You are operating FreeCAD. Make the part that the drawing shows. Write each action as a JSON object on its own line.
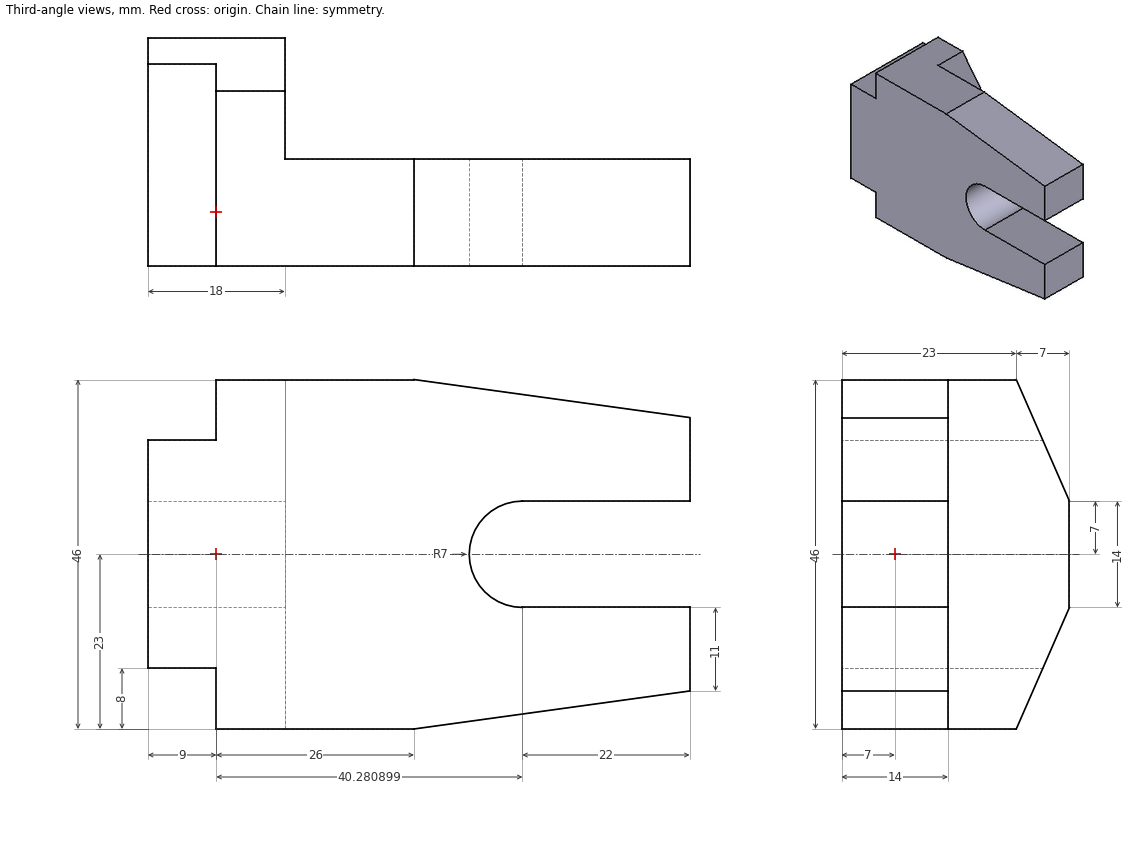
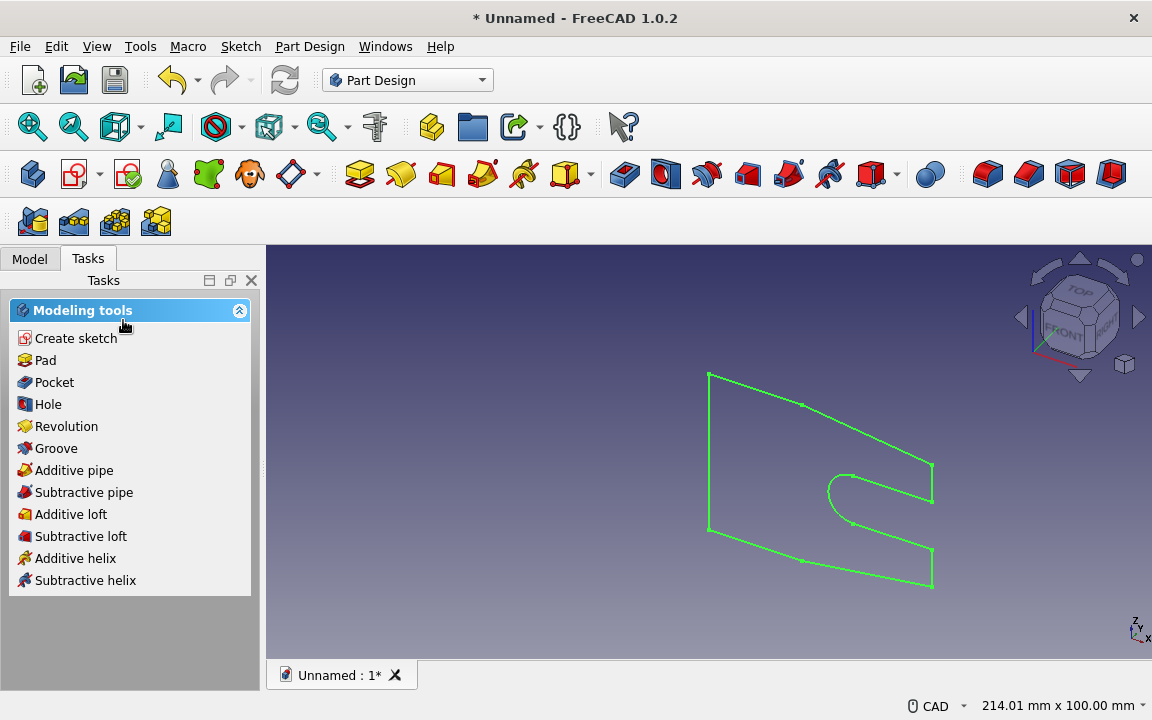
{"action": "left_click", "coordinate": [360, 174]}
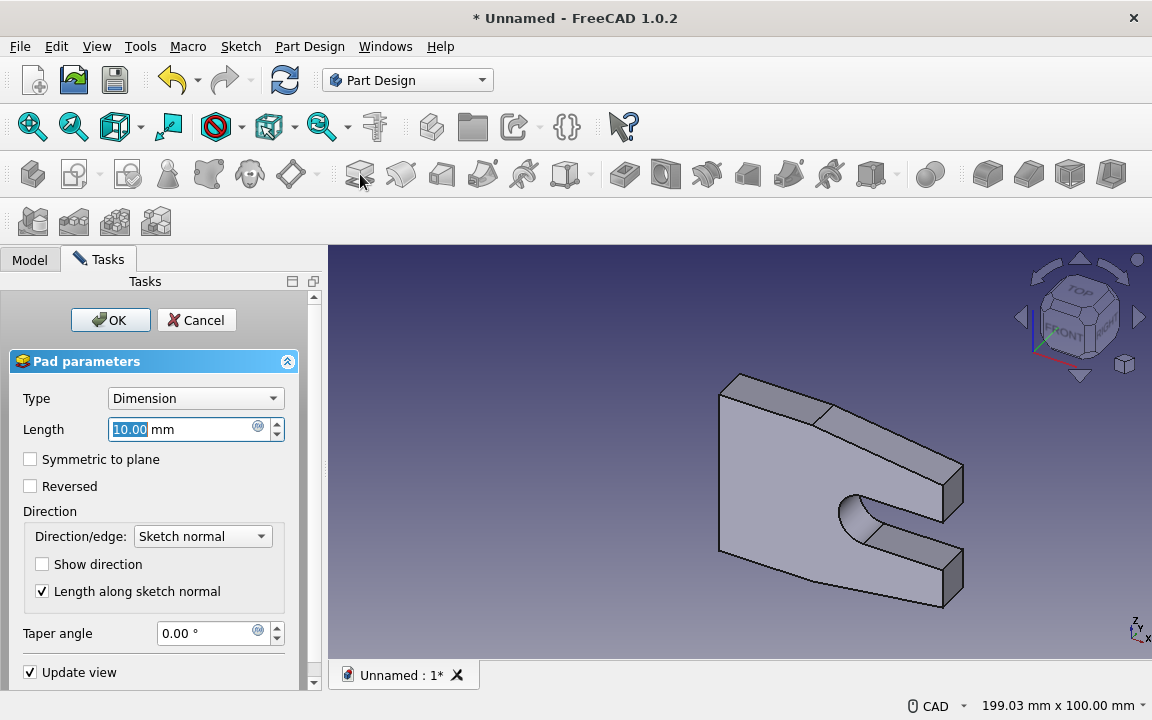
{"action": "type", "text": "14"}
{"action": "key", "text": "Tab"}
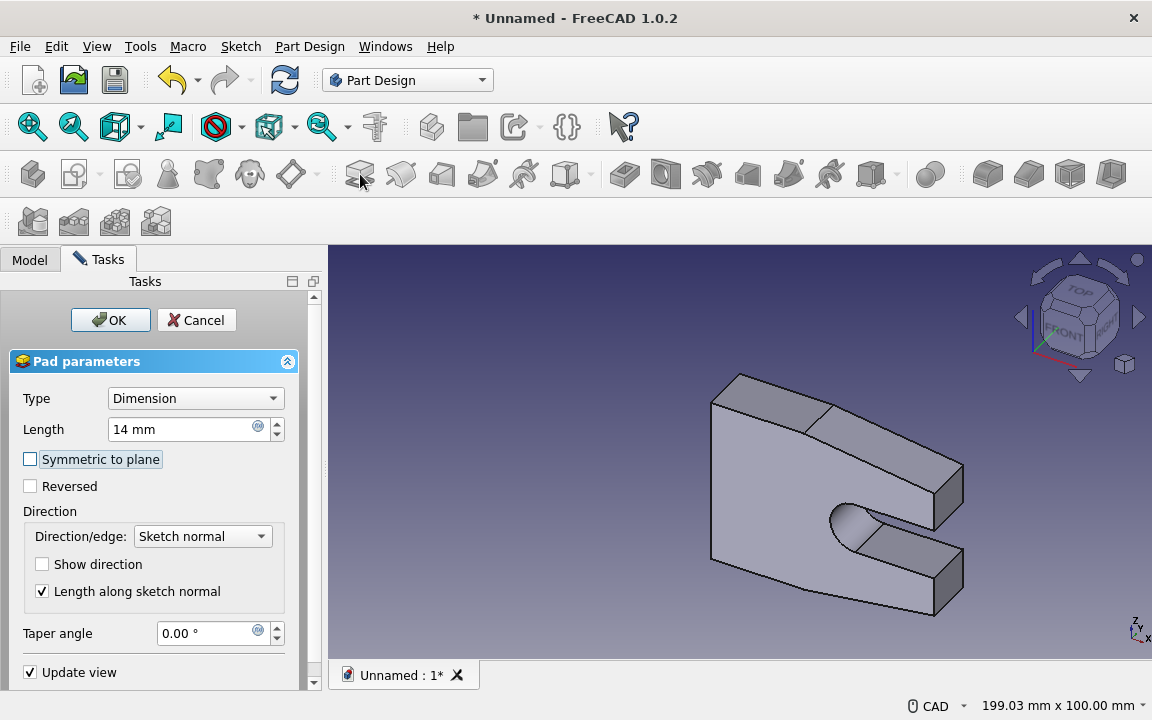
{"action": "left_click", "coordinate": [31, 459]}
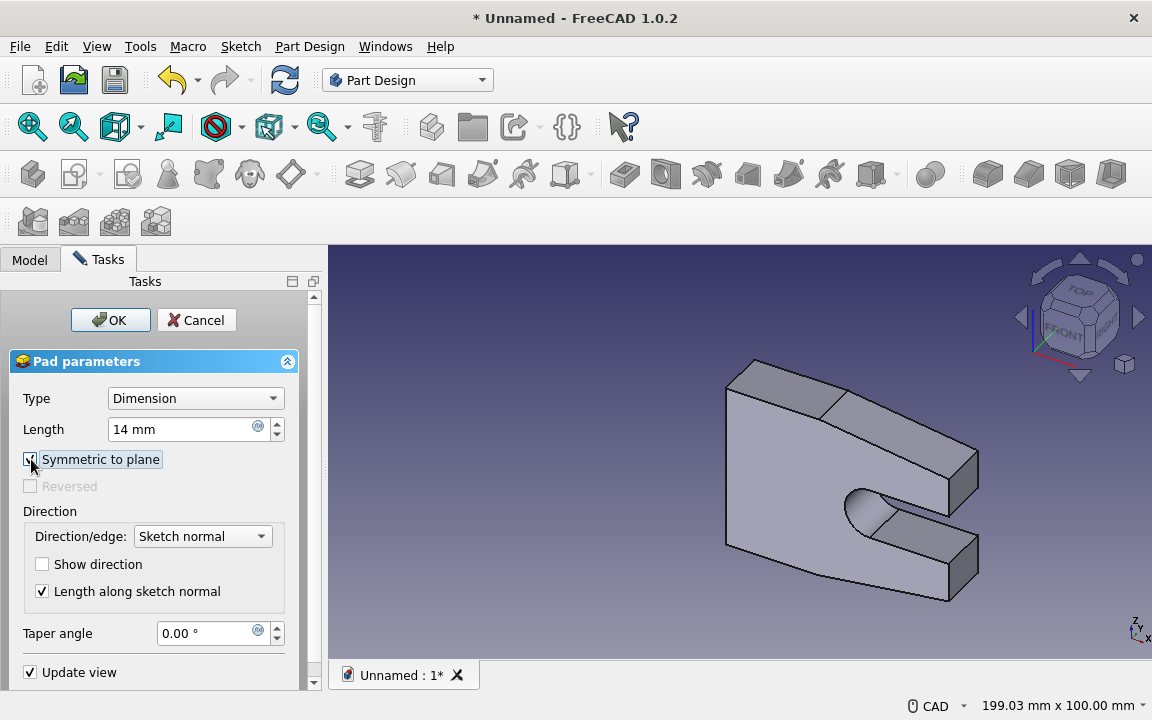
{"action": "left_click", "coordinate": [111, 320]}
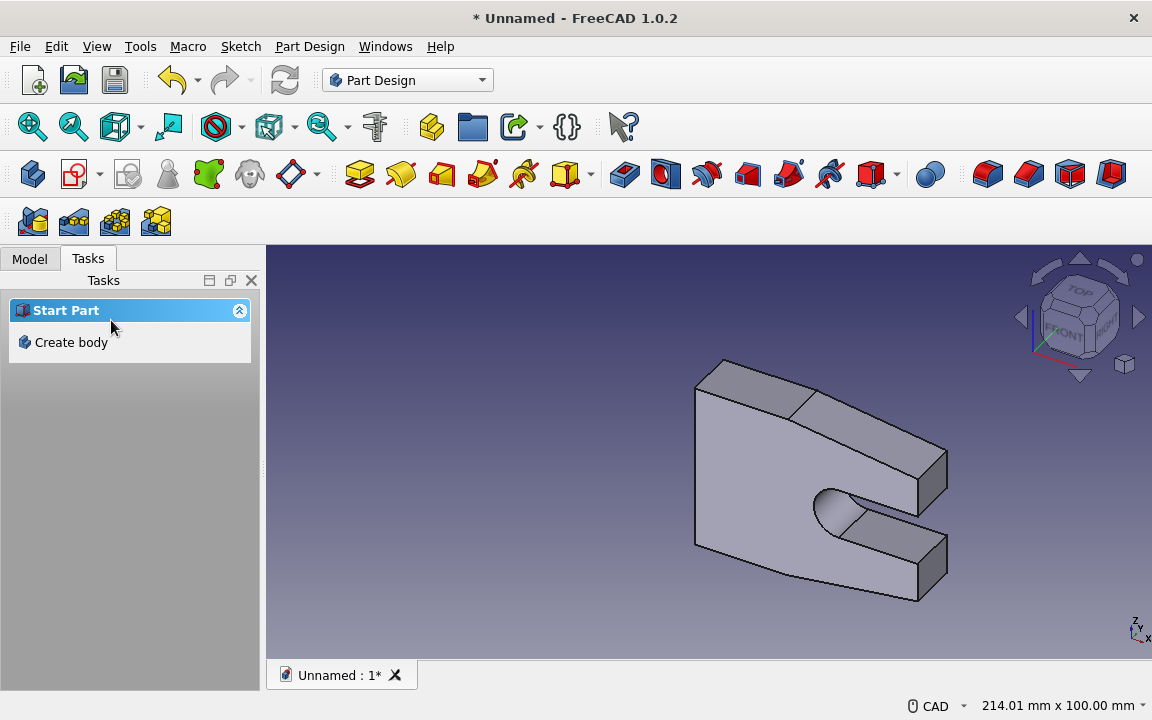
{"action": "left_click", "coordinate": [74, 174]}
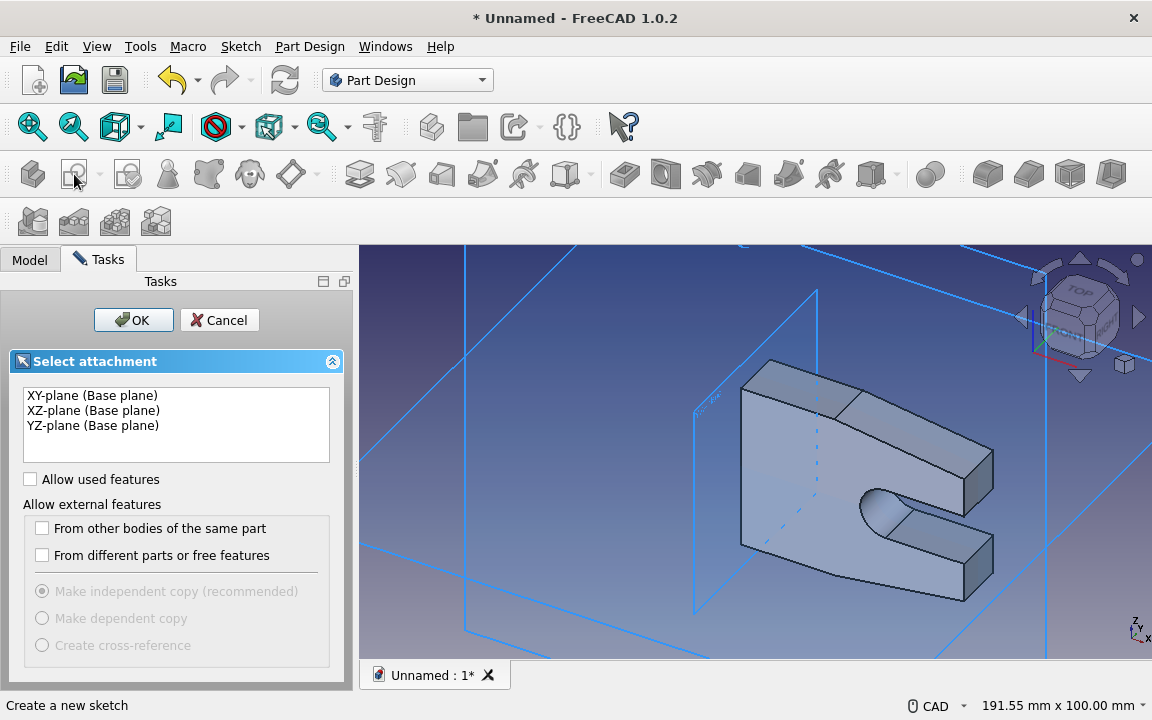
{"action": "left_click", "coordinate": [84, 426]}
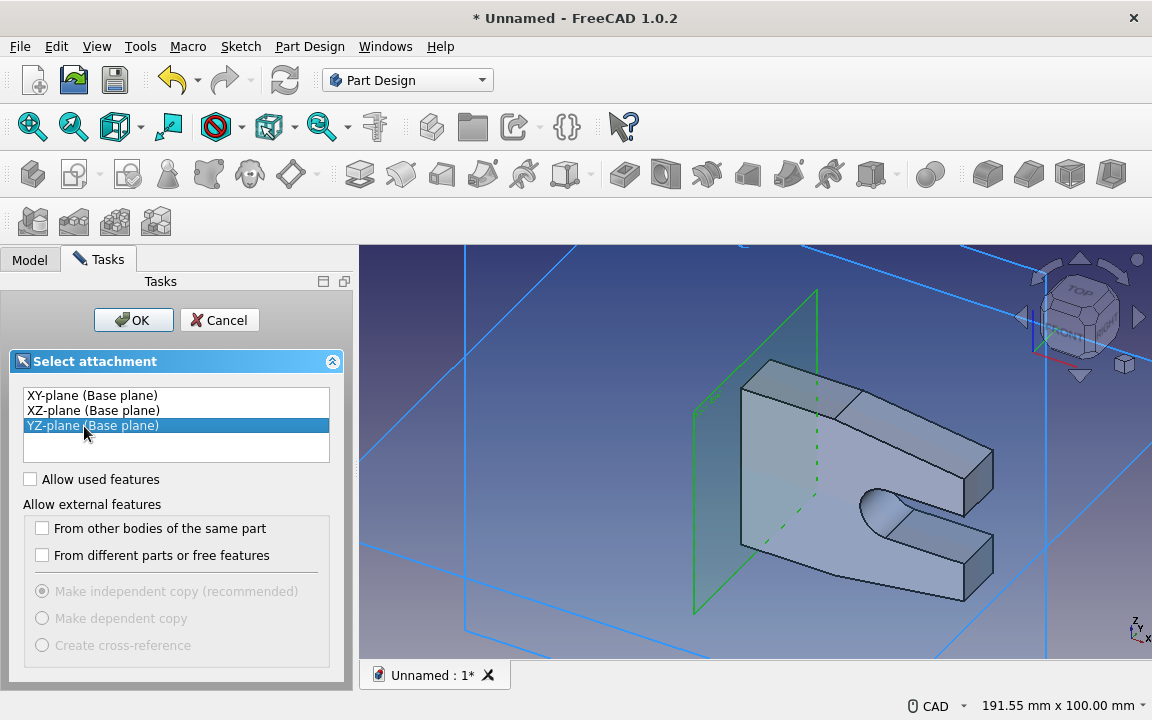
{"action": "left_click", "coordinate": [134, 320]}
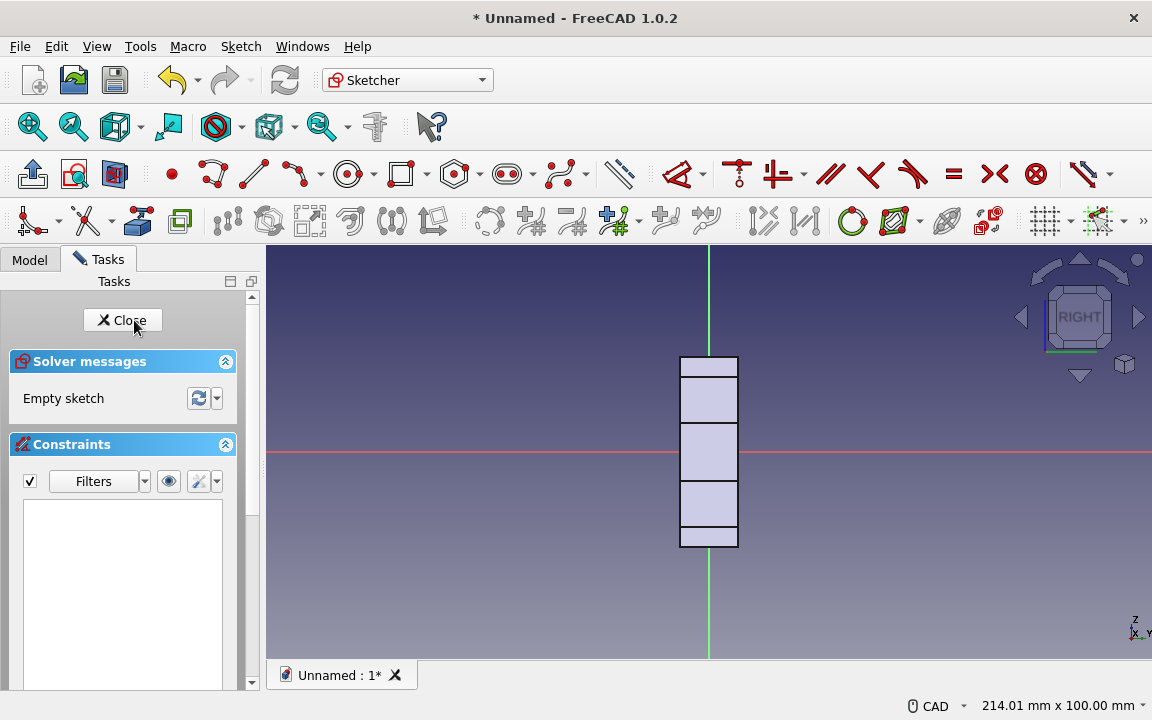
{"action": "key", "text": "q s"}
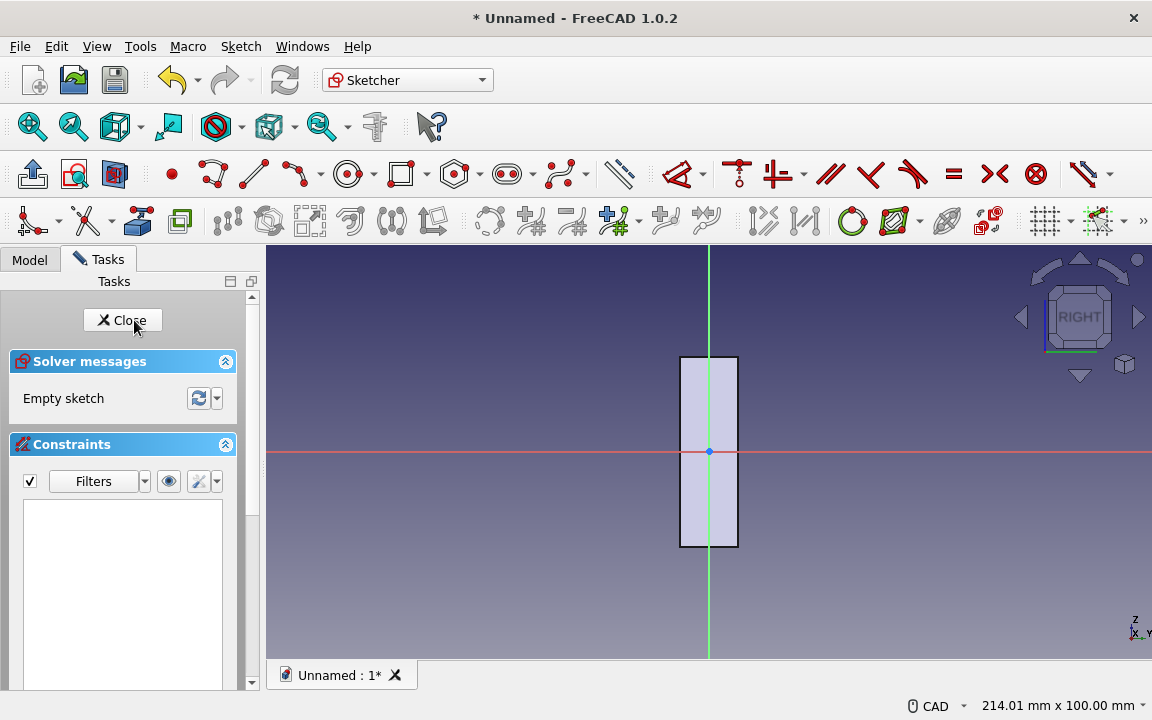
{"action": "left_click", "coordinate": [213, 174]}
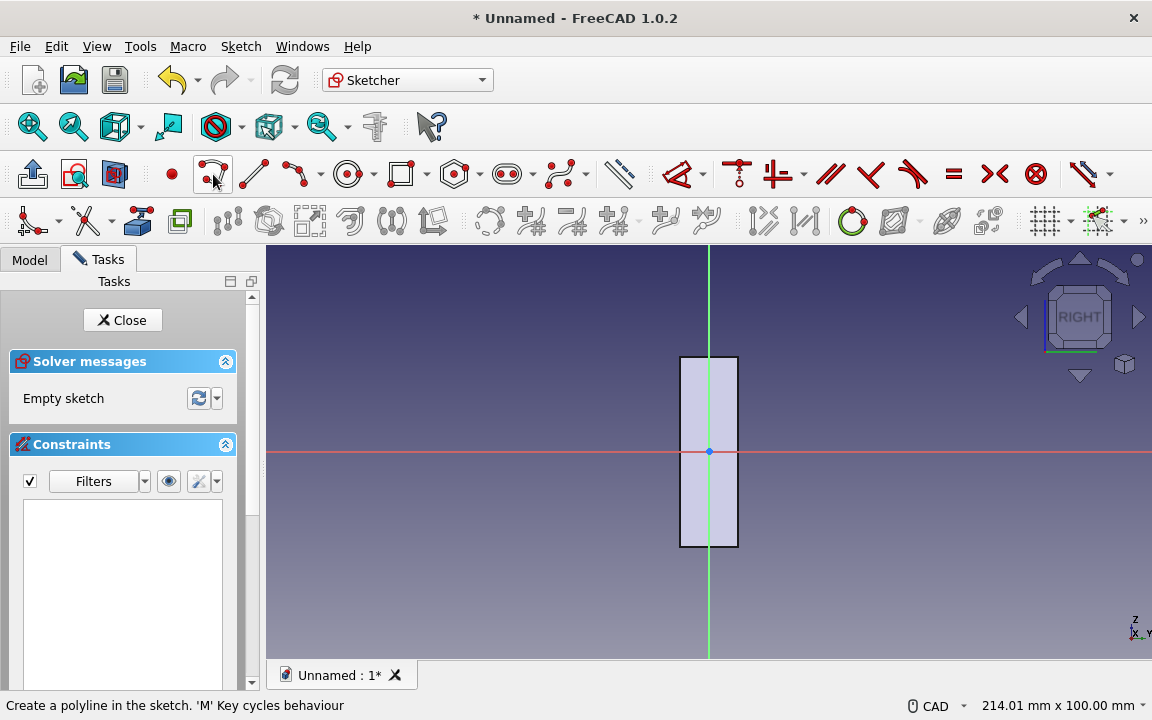
{"action": "left_click", "coordinate": [680, 547]}
{"action": "left_click", "coordinate": [680, 357]}
{"action": "left_click", "coordinate": [775, 357]}
{"action": "left_click", "coordinate": [804, 423]}
{"action": "left_click", "coordinate": [804, 481]}
{"action": "left_click", "coordinate": [775, 547]}
{"action": "left_click", "coordinate": [680, 548]}
{"action": "key", "text": "Escape"}
{"action": "key", "text": "Escape"}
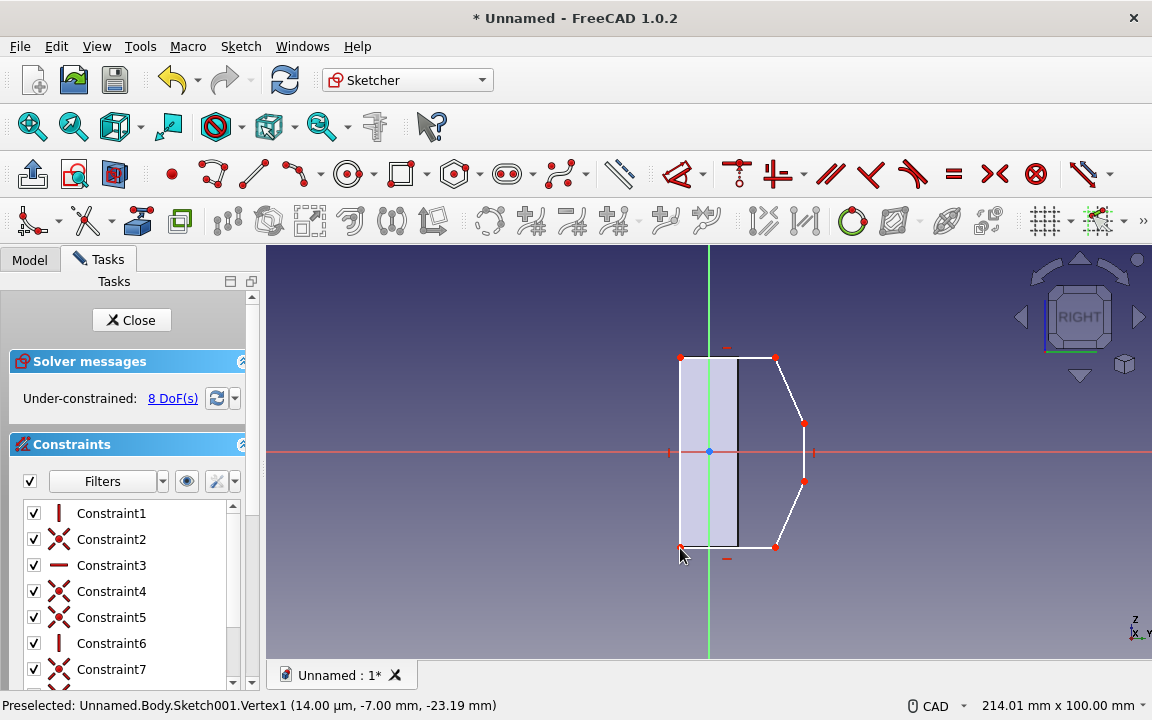
{"action": "left_click", "coordinate": [775, 358]}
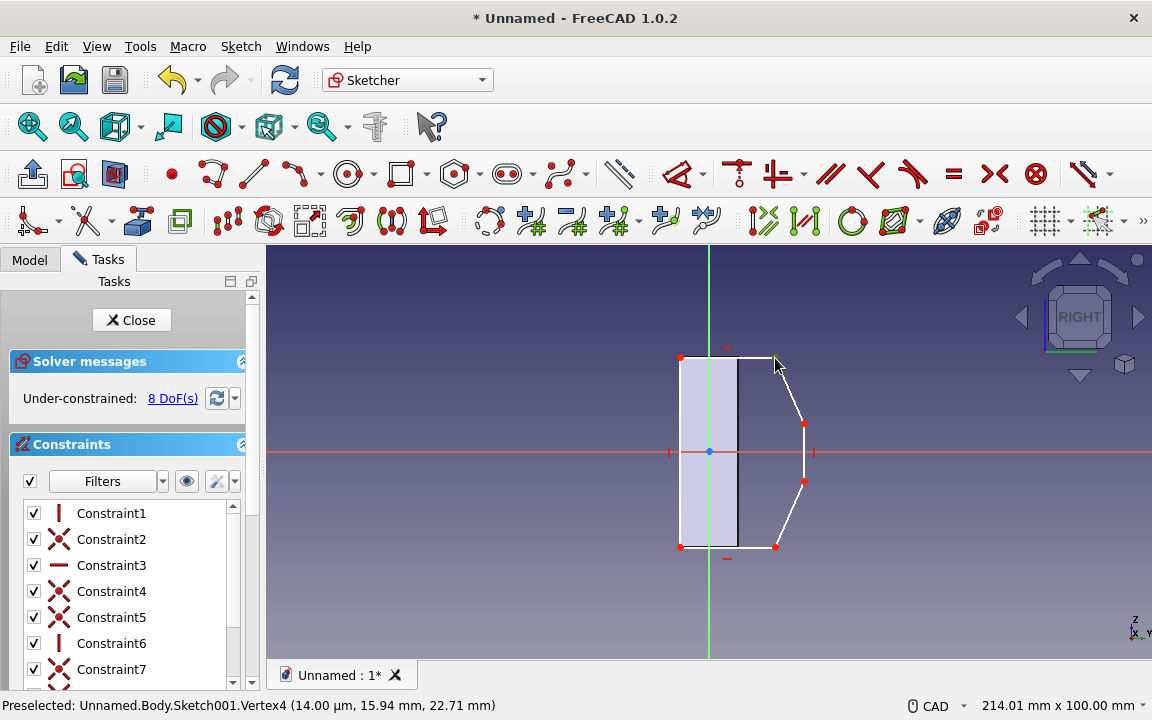
{"action": "left_click", "coordinate": [775, 548]}